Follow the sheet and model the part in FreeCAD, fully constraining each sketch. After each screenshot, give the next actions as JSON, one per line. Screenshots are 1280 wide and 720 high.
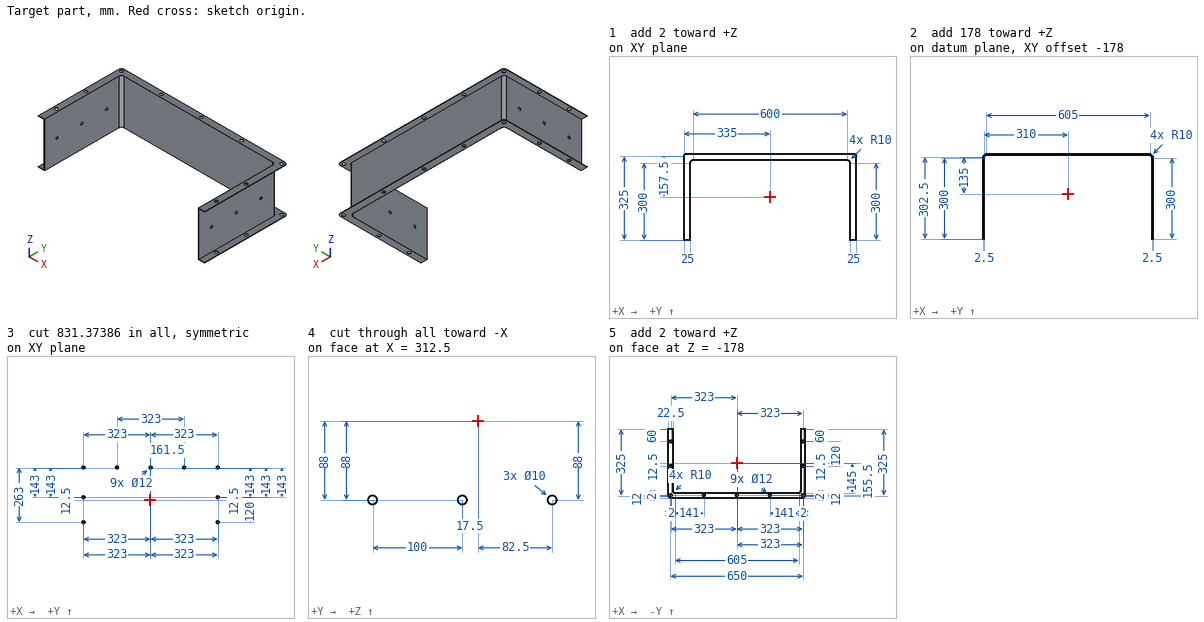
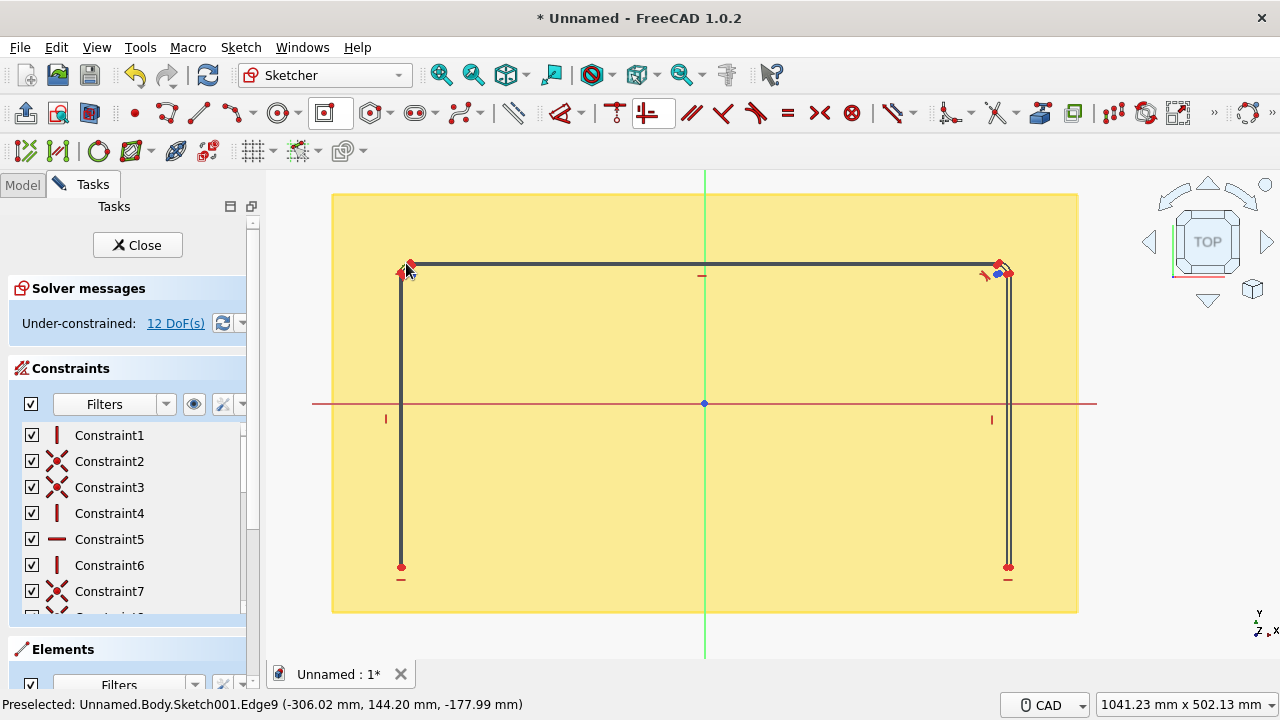
{"action": "scroll", "coordinate": [1009, 269], "scroll_direction": "up", "scroll_amount": 7}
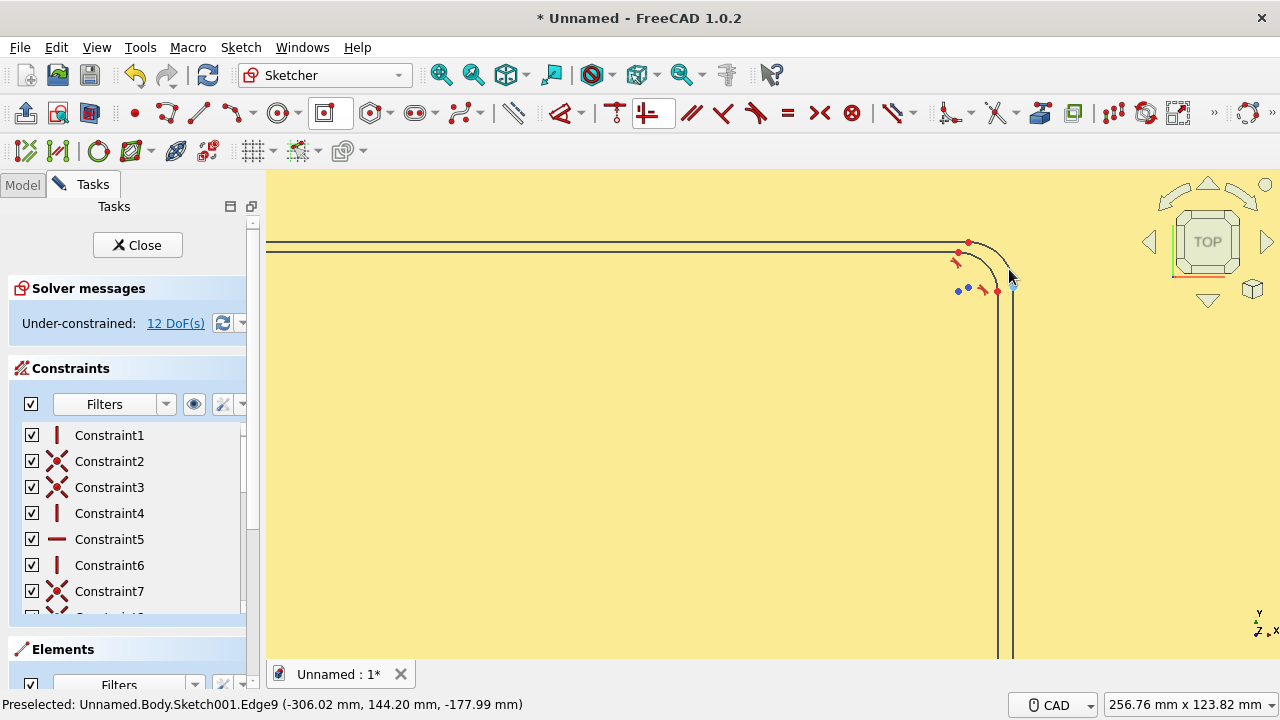
{"action": "left_click", "coordinate": [1008, 267]}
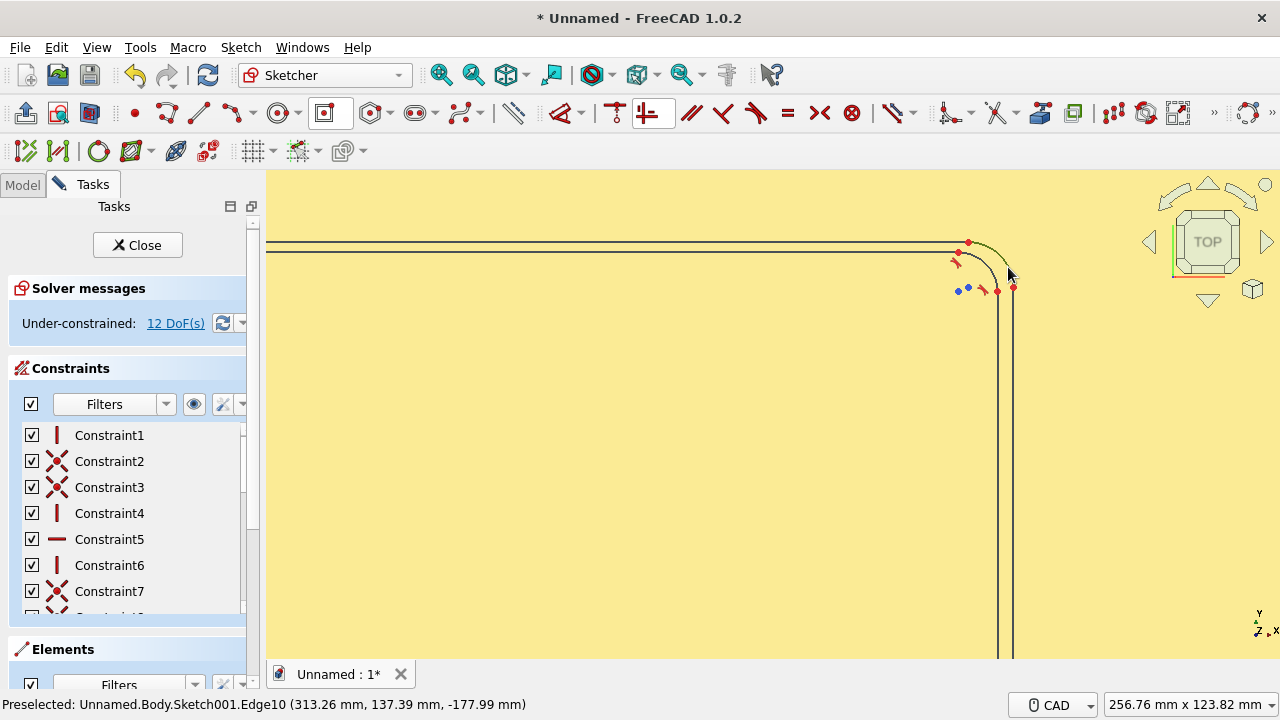
{"action": "left_click", "coordinate": [993, 274]}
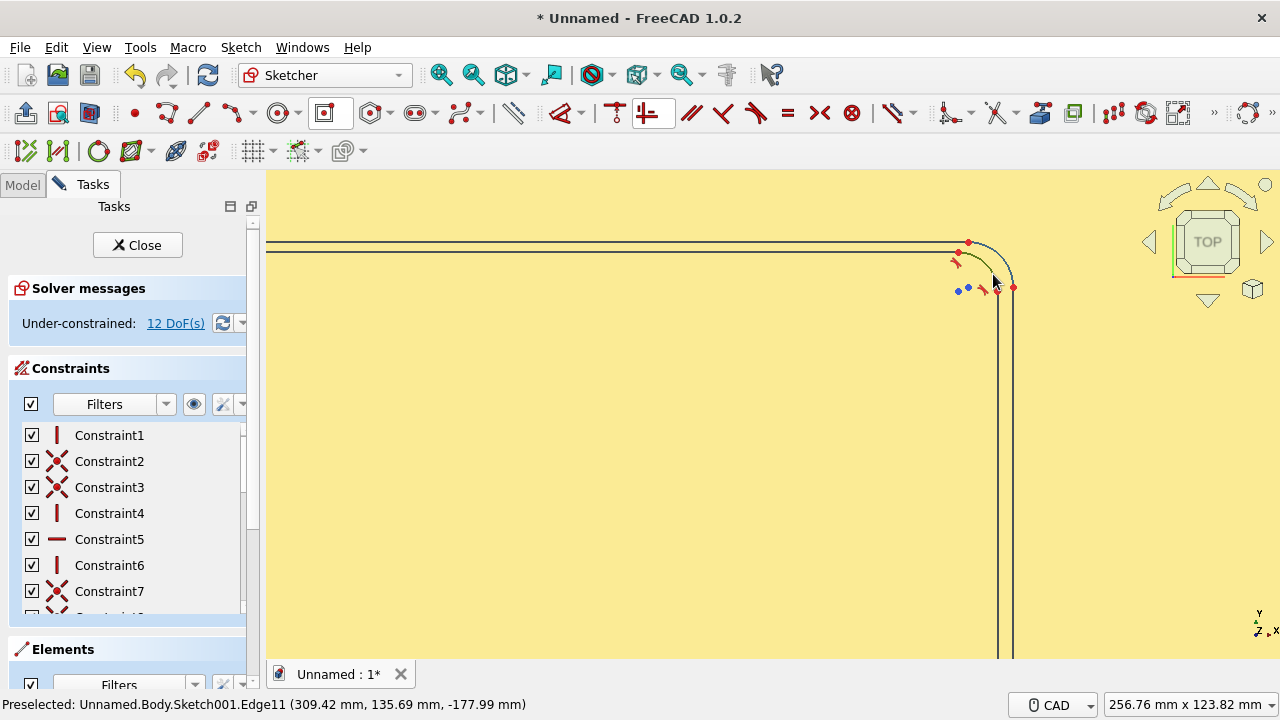
{"action": "scroll", "coordinate": [1009, 269], "scroll_direction": "down", "scroll_amount": 7}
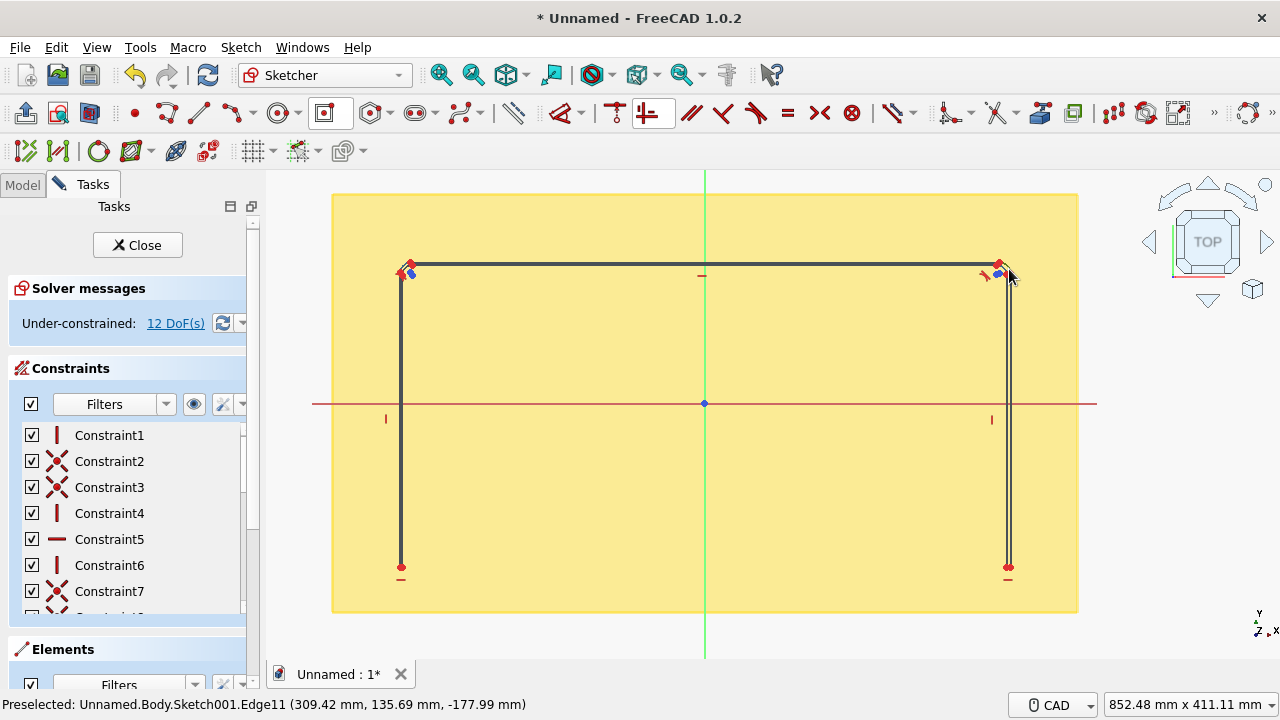
{"action": "scroll", "coordinate": [408, 266], "scroll_direction": "up", "scroll_amount": 8}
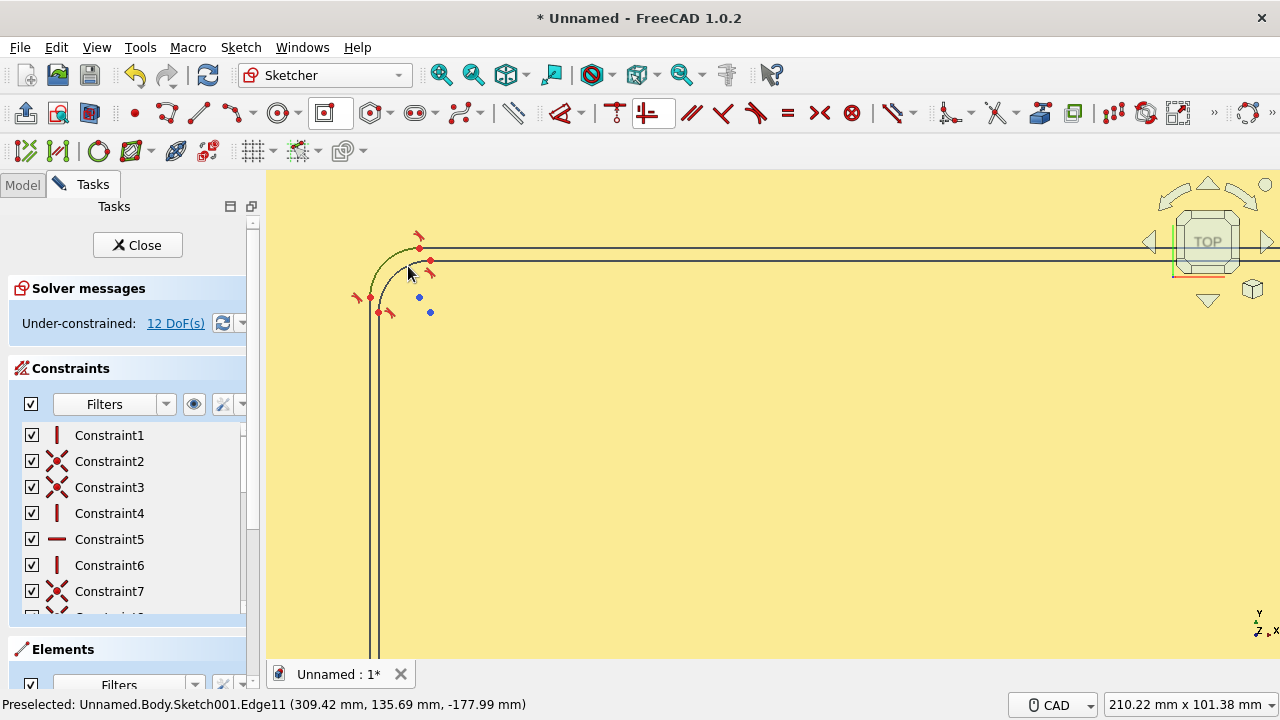
{"action": "left_click", "coordinate": [407, 266]}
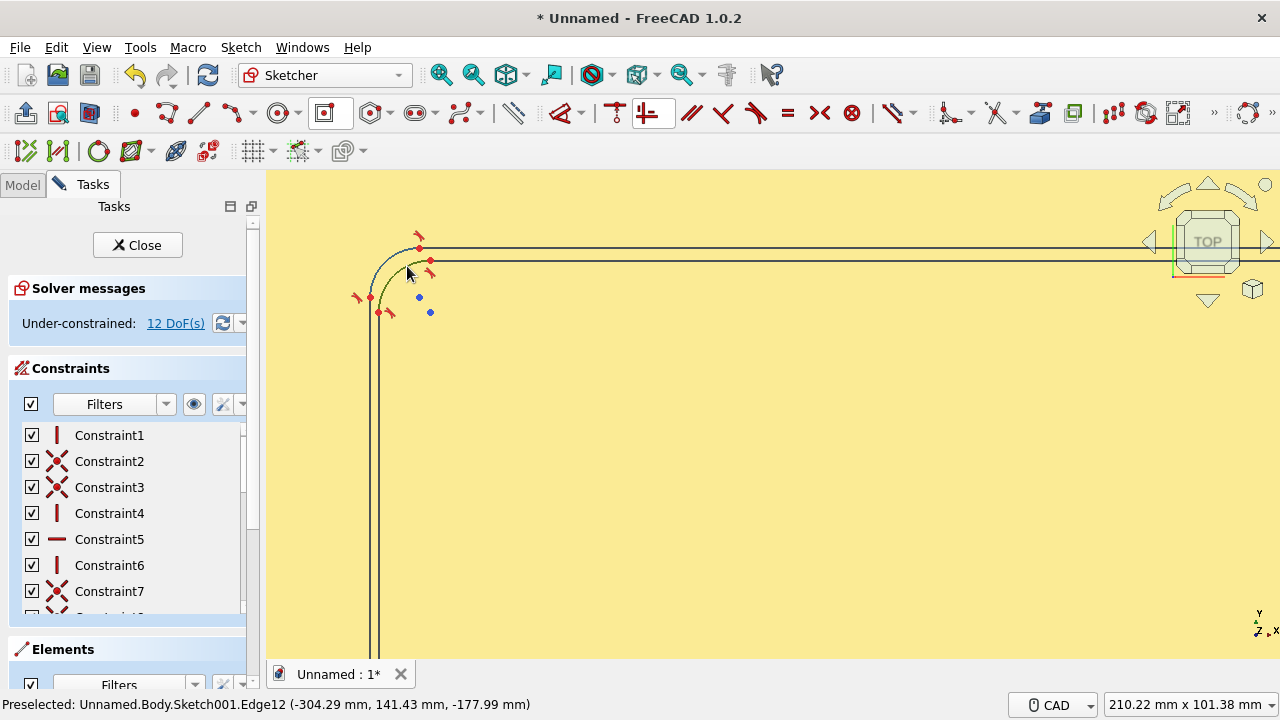
{"action": "key", "text": "e"}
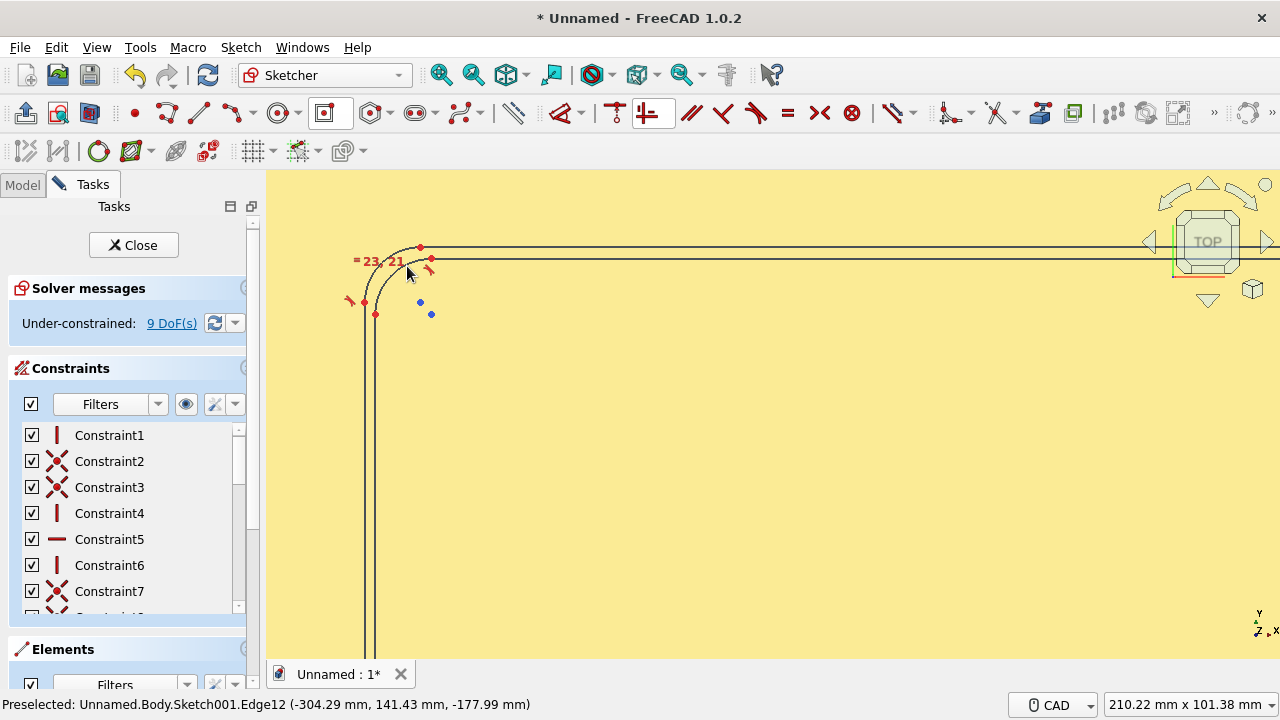
{"action": "left_click", "coordinate": [560, 114]}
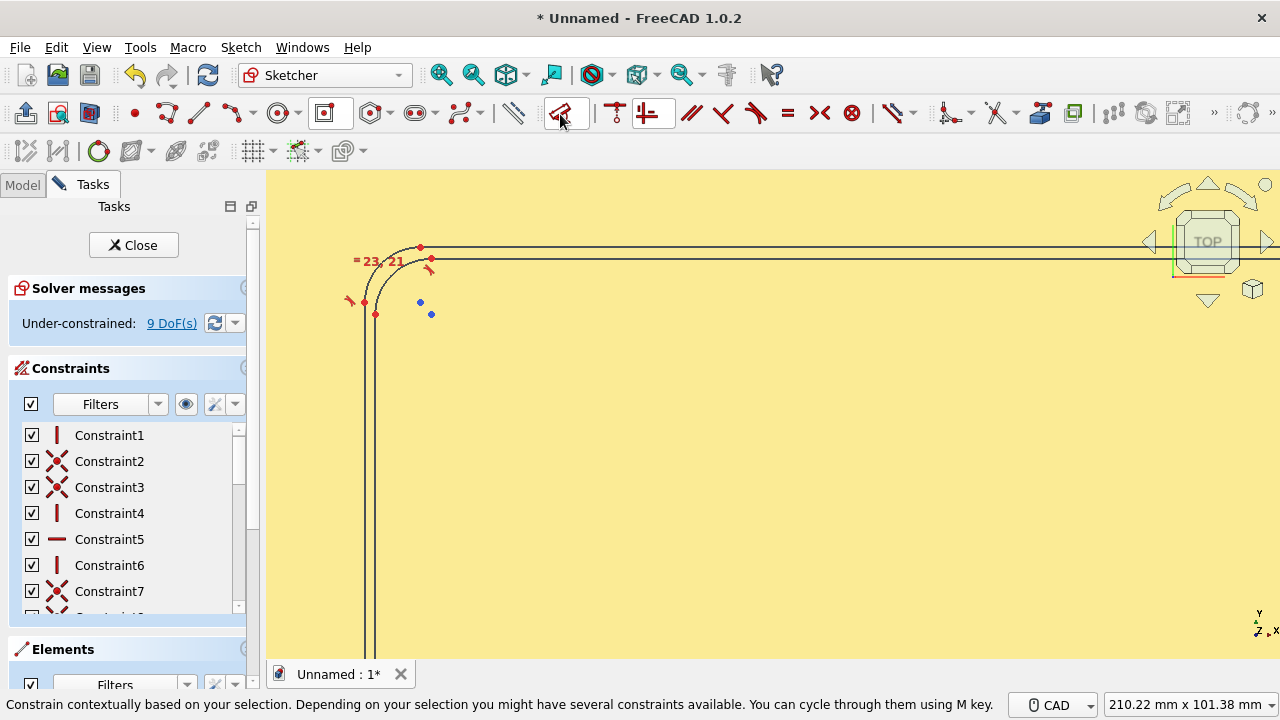
{"action": "left_click", "coordinate": [395, 253]}
{"action": "left_click", "coordinate": [380, 225]}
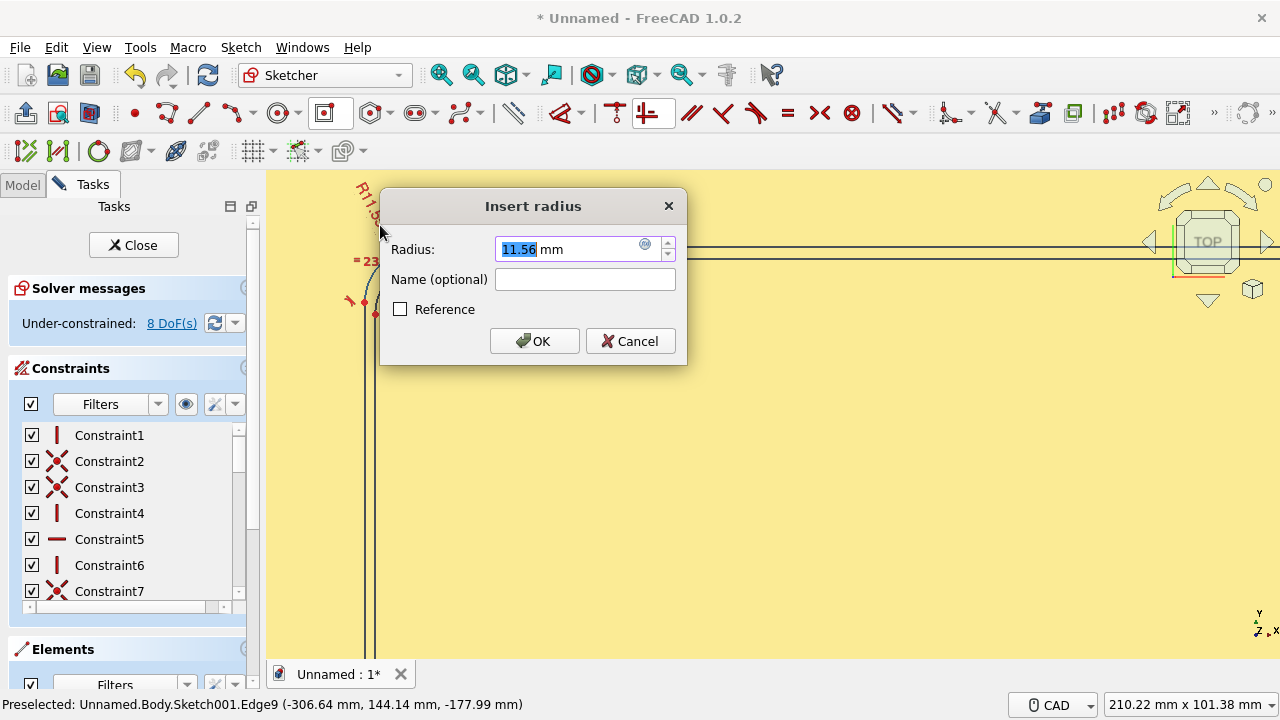
{"action": "type", "text": "10"}
{"action": "key", "text": "Return"}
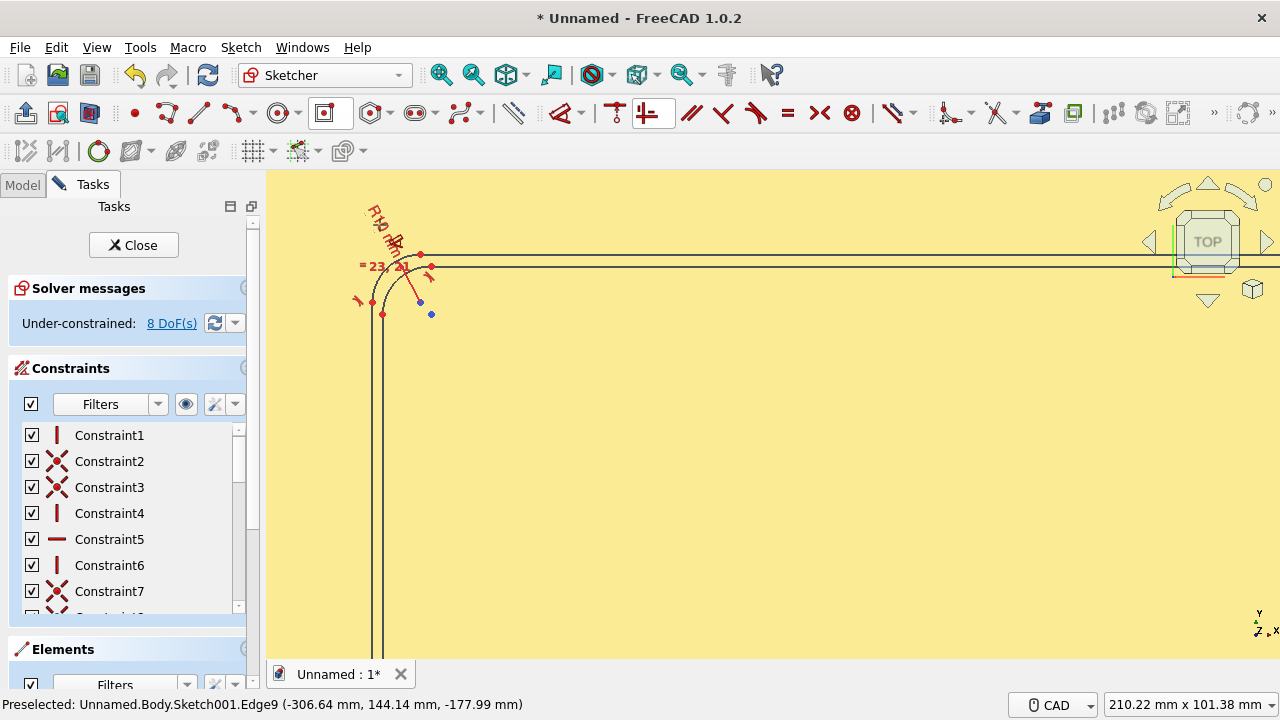
{"action": "scroll", "coordinate": [383, 604], "scroll_direction": "up", "scroll_amount": 2}